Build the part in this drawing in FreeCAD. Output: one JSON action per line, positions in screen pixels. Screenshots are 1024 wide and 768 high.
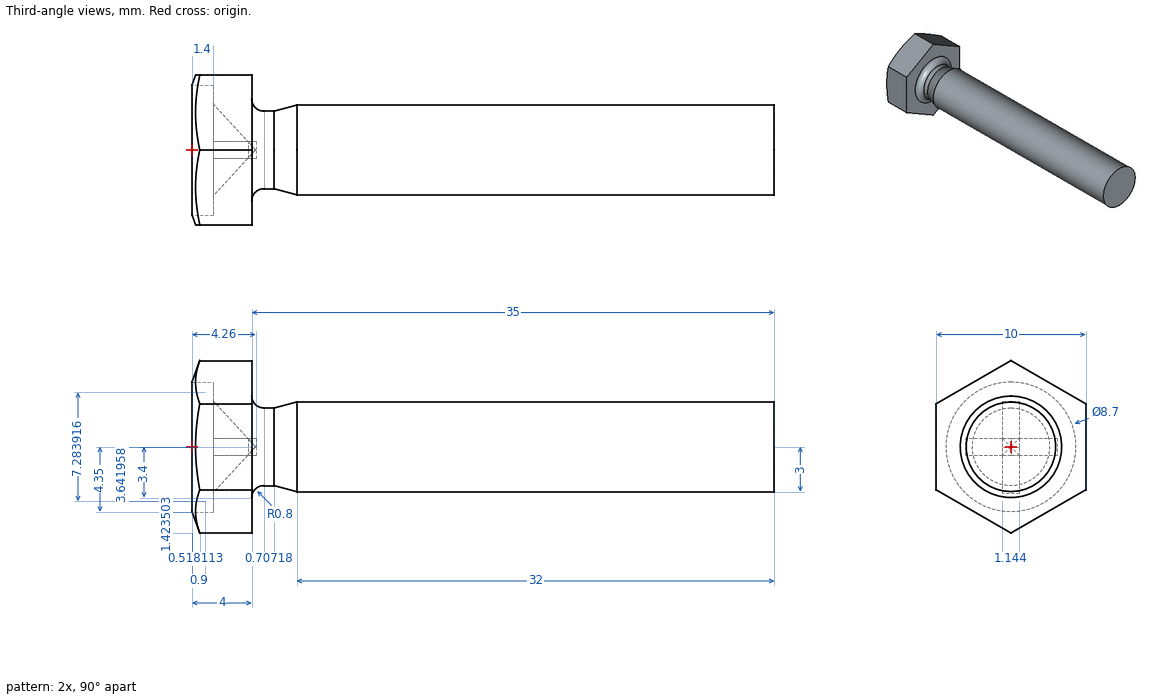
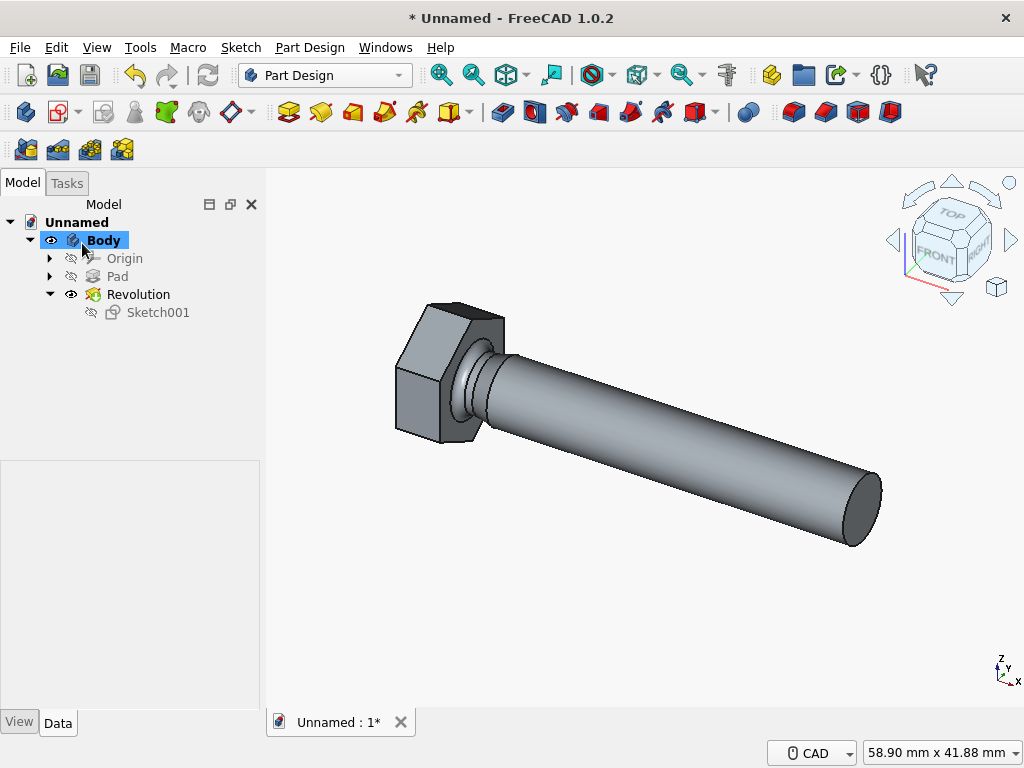
{"action": "left_click", "coordinate": [58, 112]}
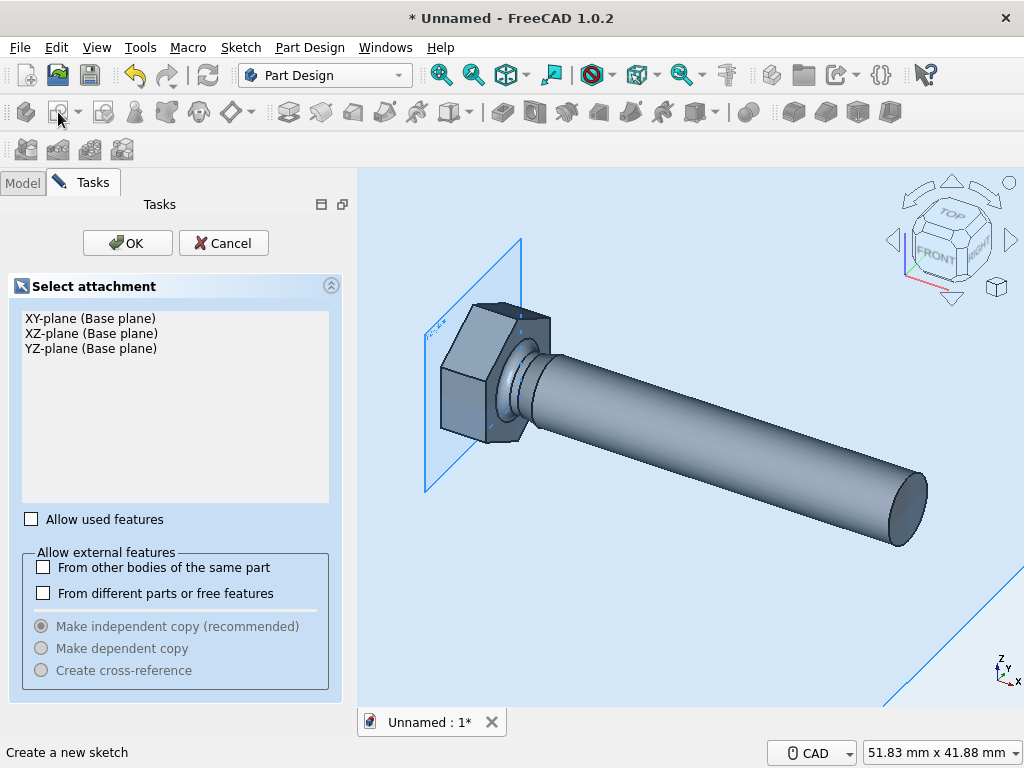
{"action": "left_click", "coordinate": [82, 334]}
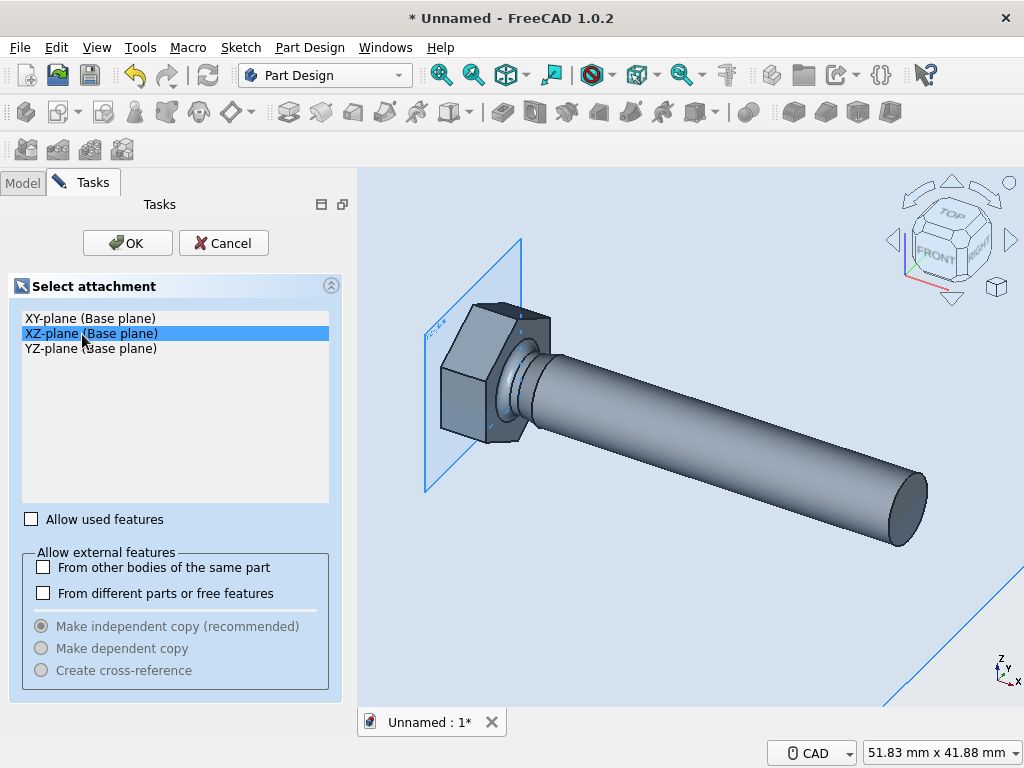
{"action": "left_click", "coordinate": [128, 243]}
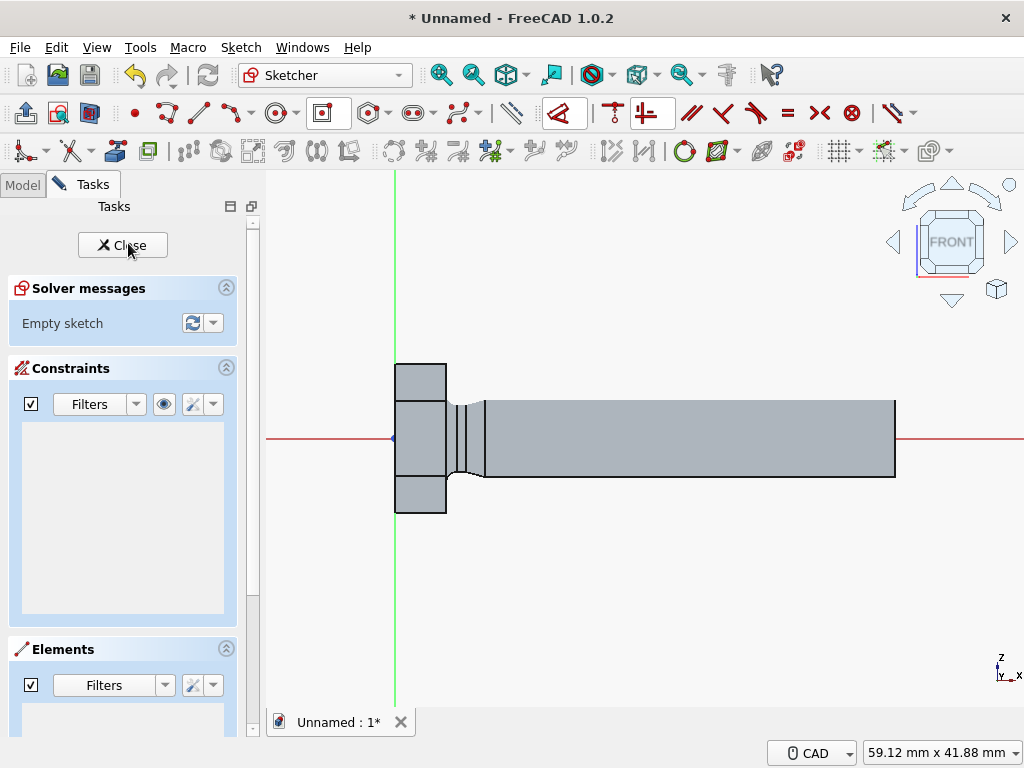
{"action": "key", "text": "q s"}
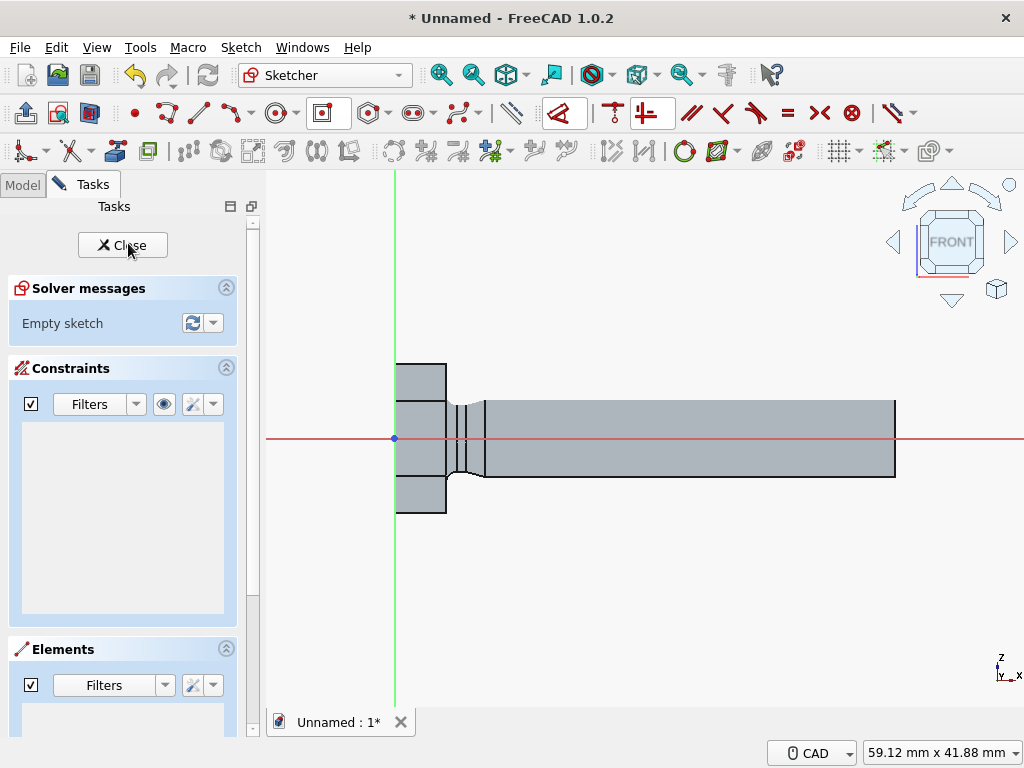
{"action": "scroll", "coordinate": [389, 507], "scroll_direction": "up", "scroll_amount": 15}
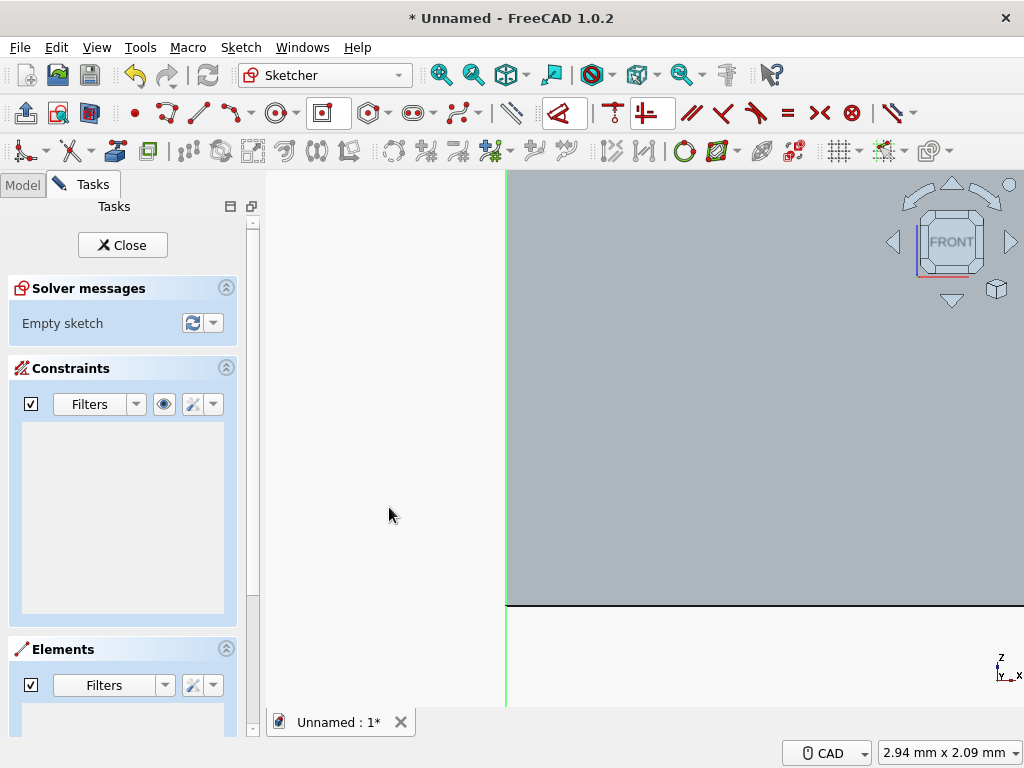
{"action": "left_click", "coordinate": [168, 114]}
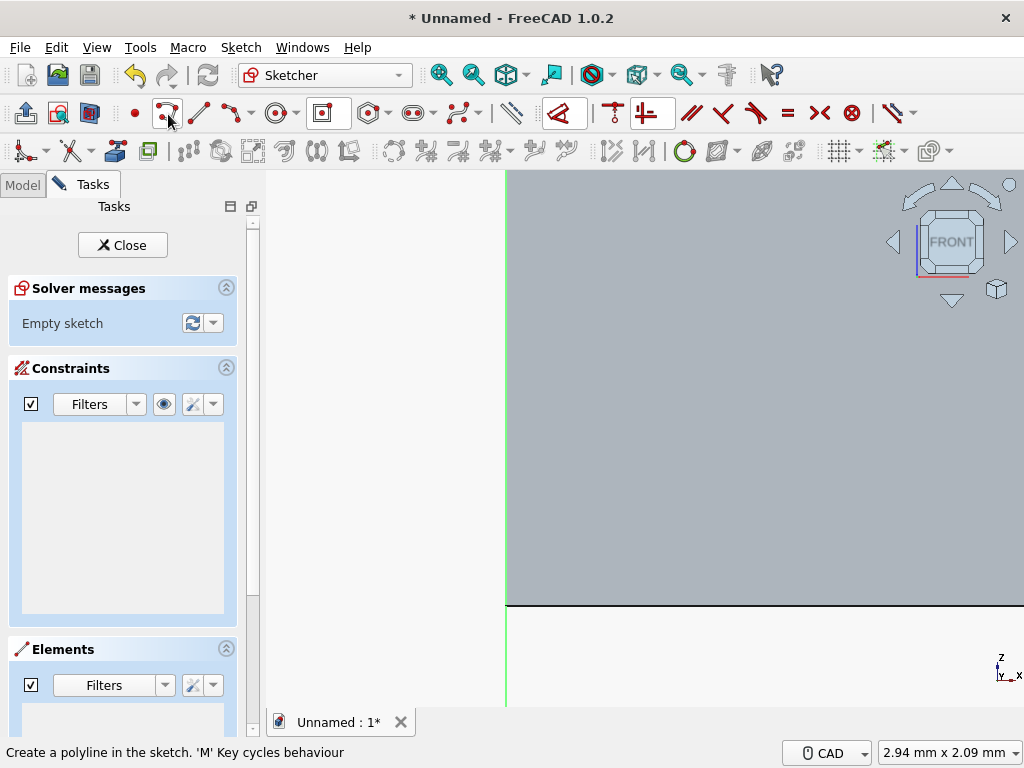
{"action": "left_click", "coordinate": [506, 239]}
{"action": "left_click", "coordinate": [640, 606]}
{"action": "left_click", "coordinate": [515, 606]}
{"action": "left_click", "coordinate": [506, 240]}
{"action": "key", "text": "Escape"}
{"action": "key", "text": "Escape"}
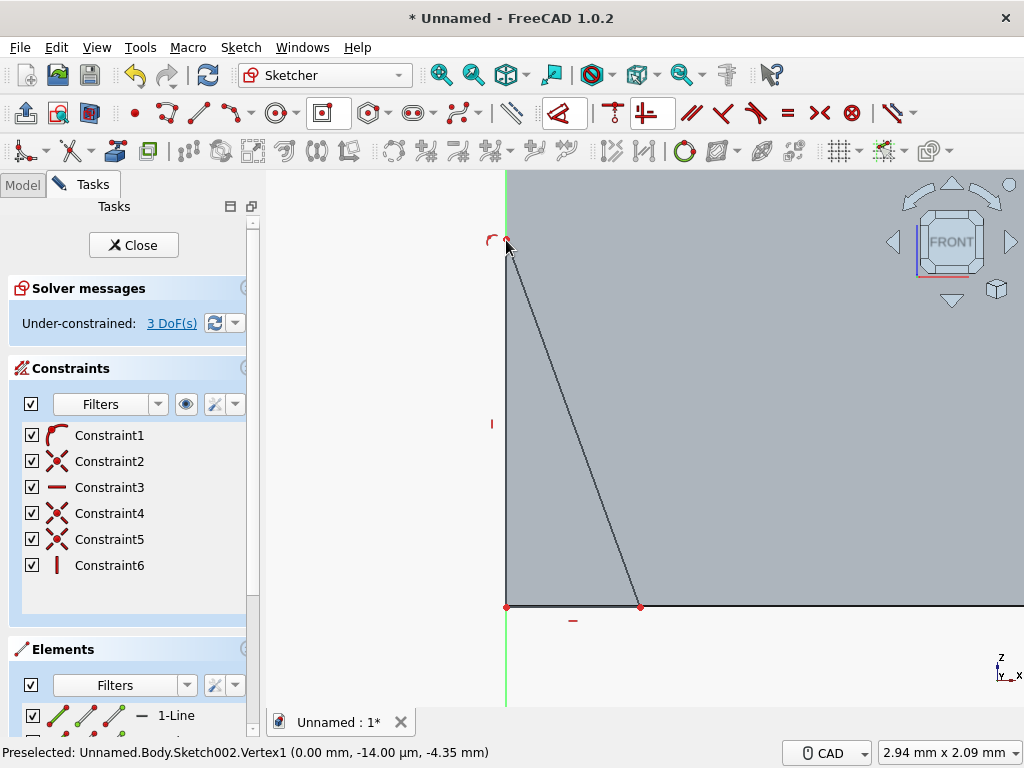
{"action": "left_click", "coordinate": [506, 240]}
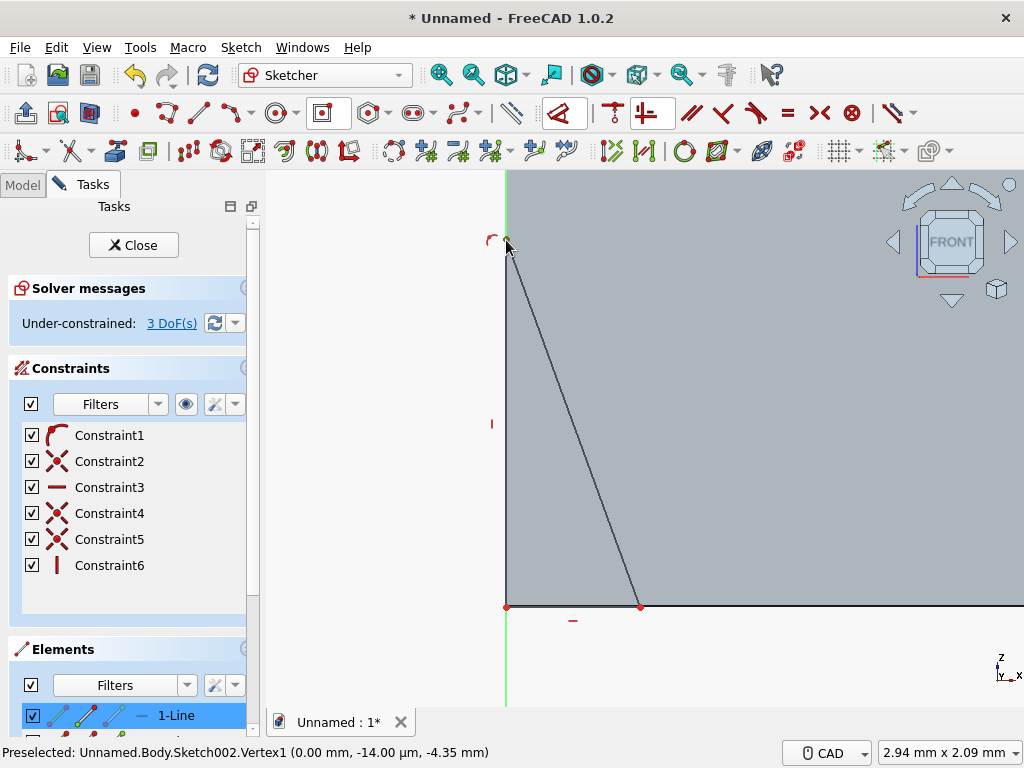
{"action": "left_click", "coordinate": [582, 114]}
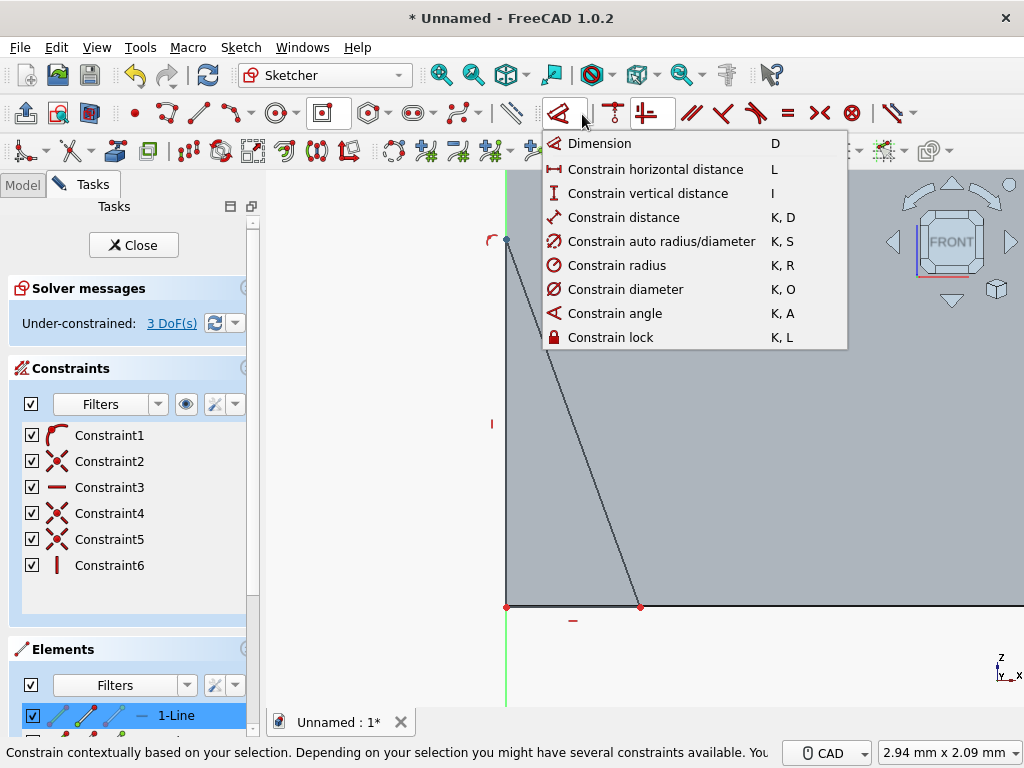
{"action": "left_click", "coordinate": [695, 193]}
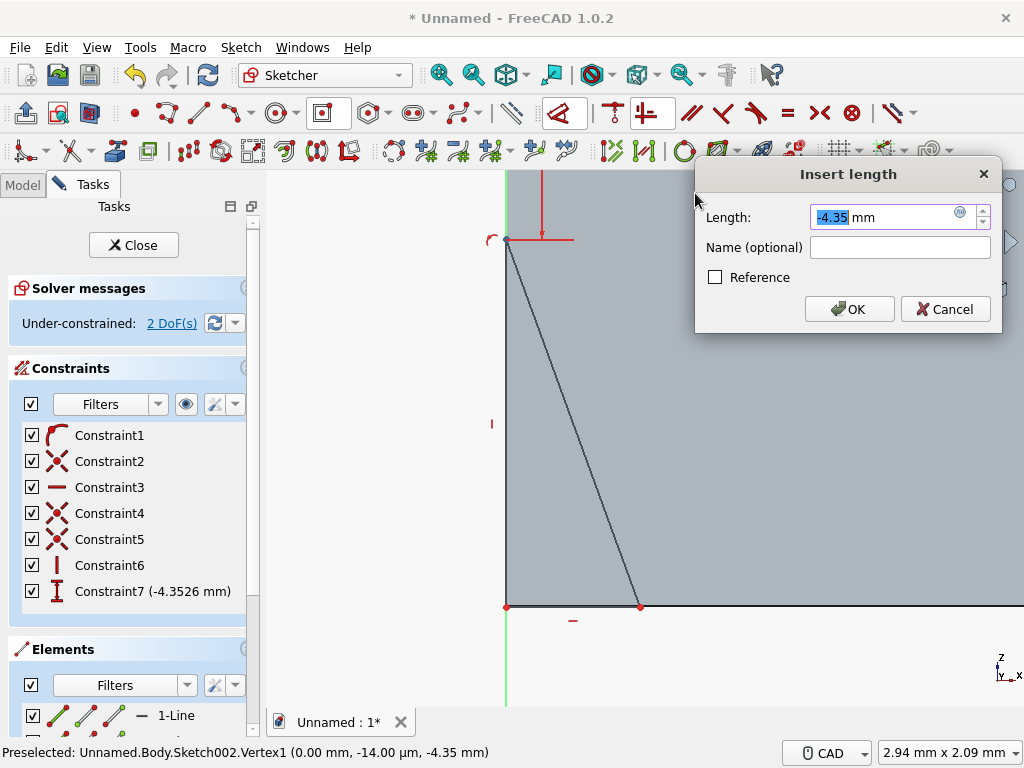
{"action": "type", "text": "-4.35"}
{"action": "key", "text": "Return"}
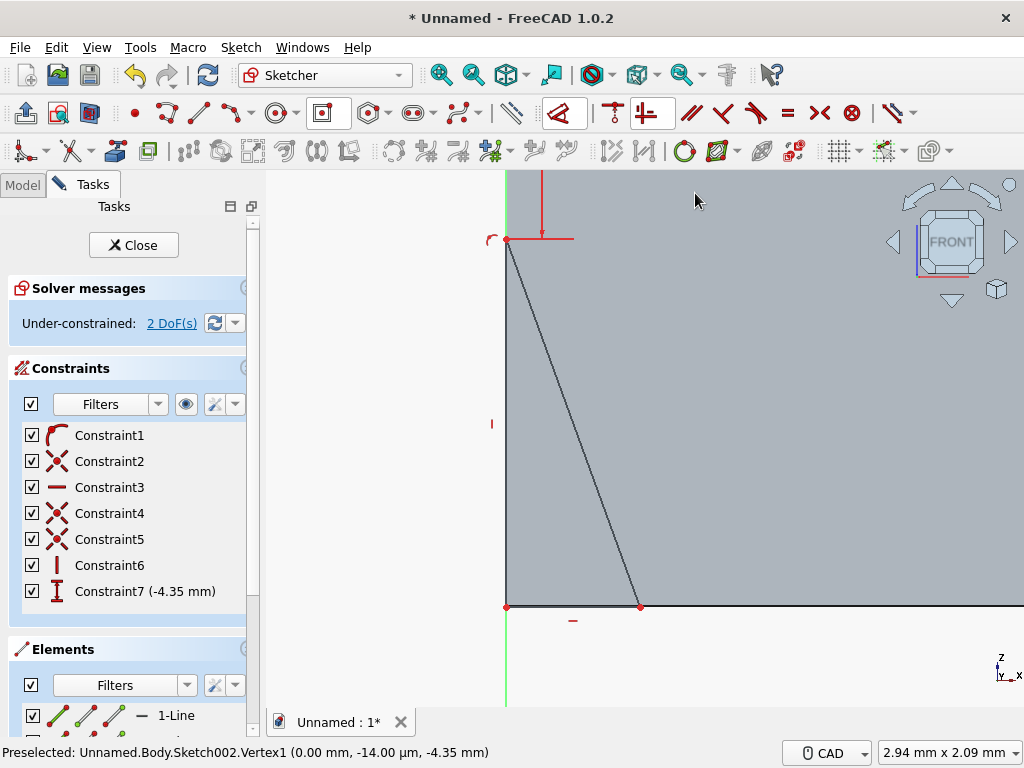
{"action": "left_click", "coordinate": [600, 607]}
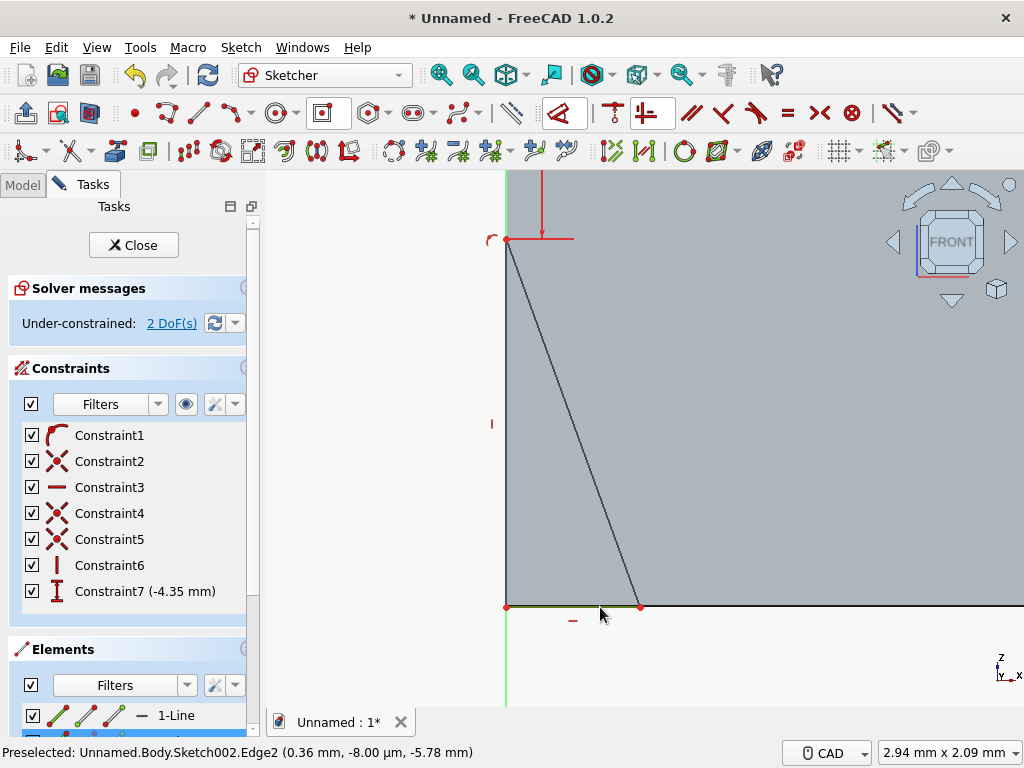
{"action": "left_click", "coordinate": [582, 114]}